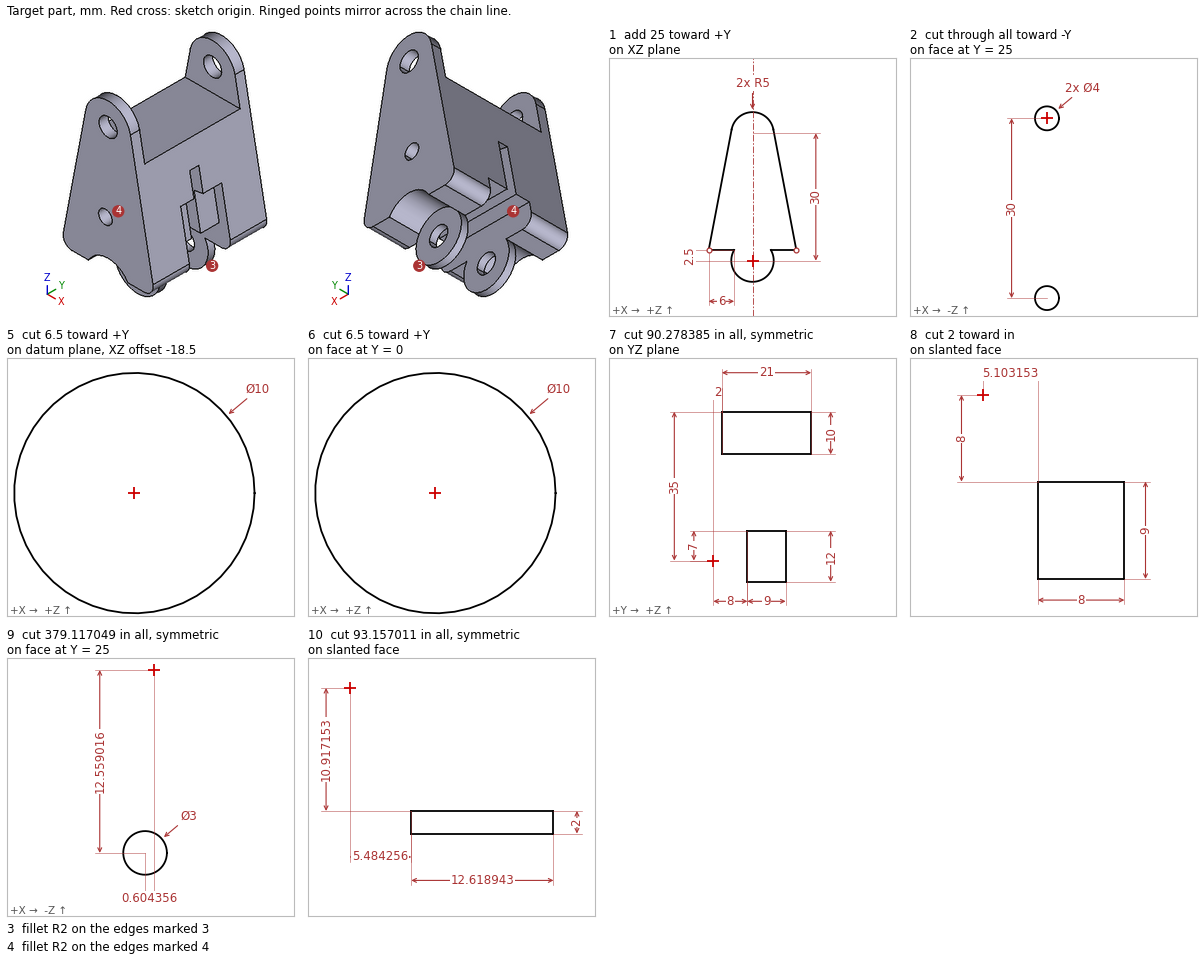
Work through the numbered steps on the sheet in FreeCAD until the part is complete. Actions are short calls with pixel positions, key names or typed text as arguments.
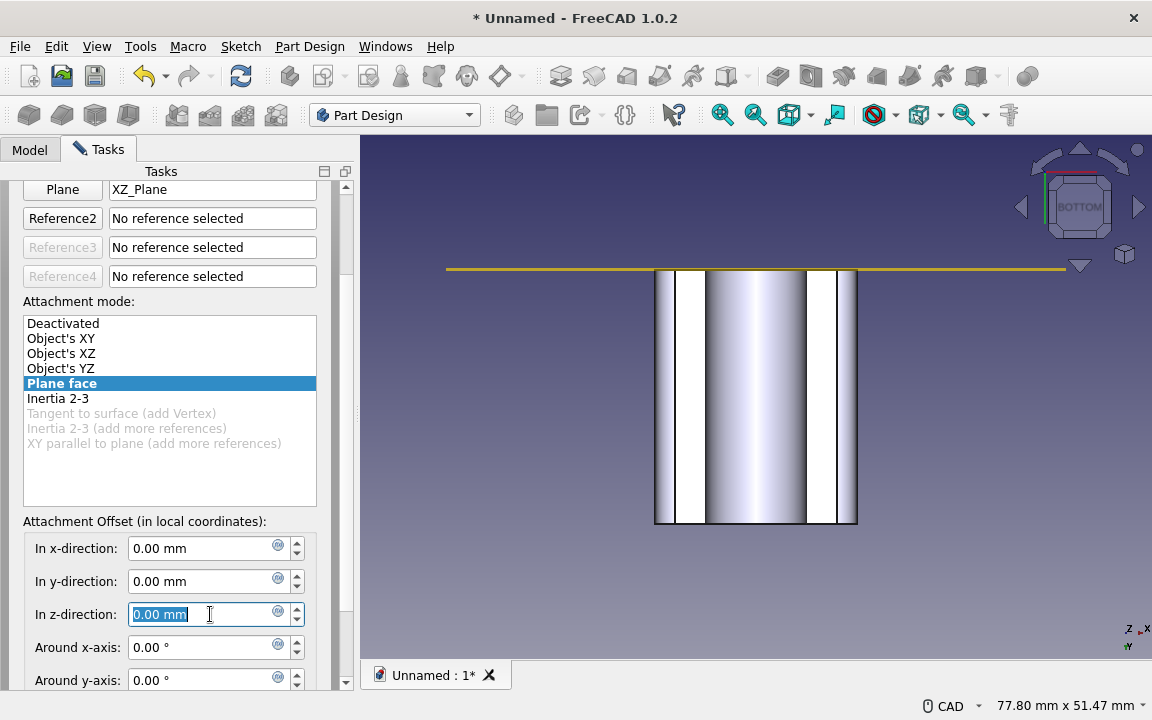
text(-18.5)
key(Tab)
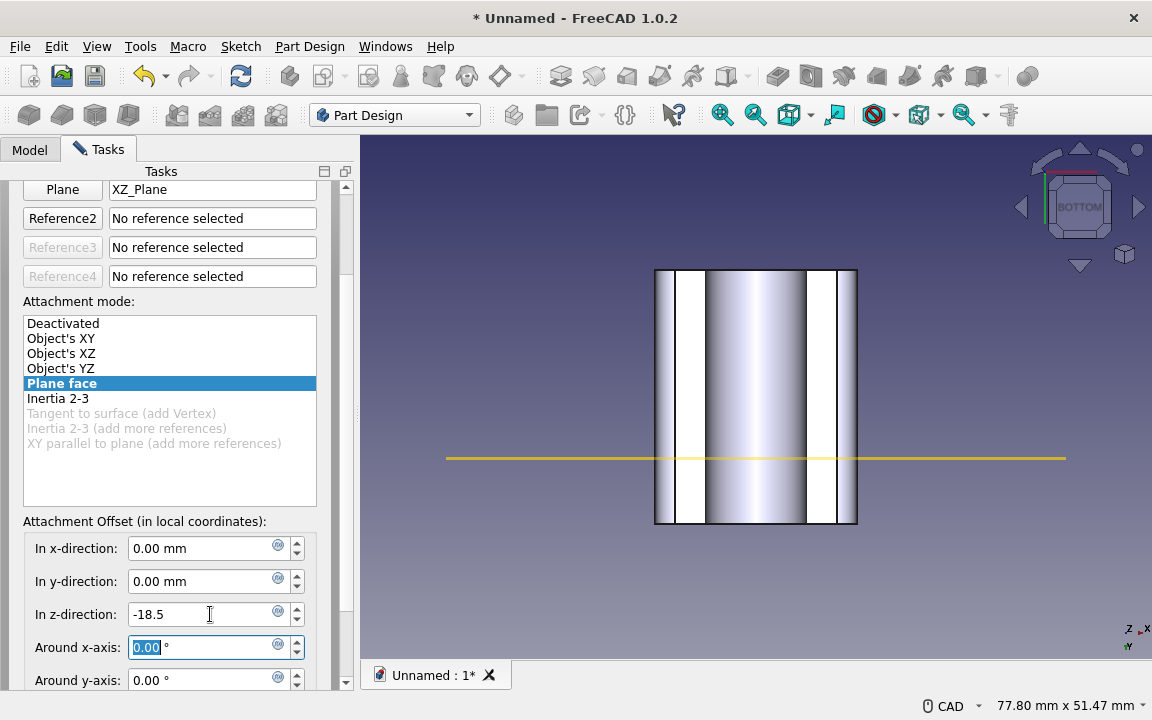
scroll(346, 436, up, 3)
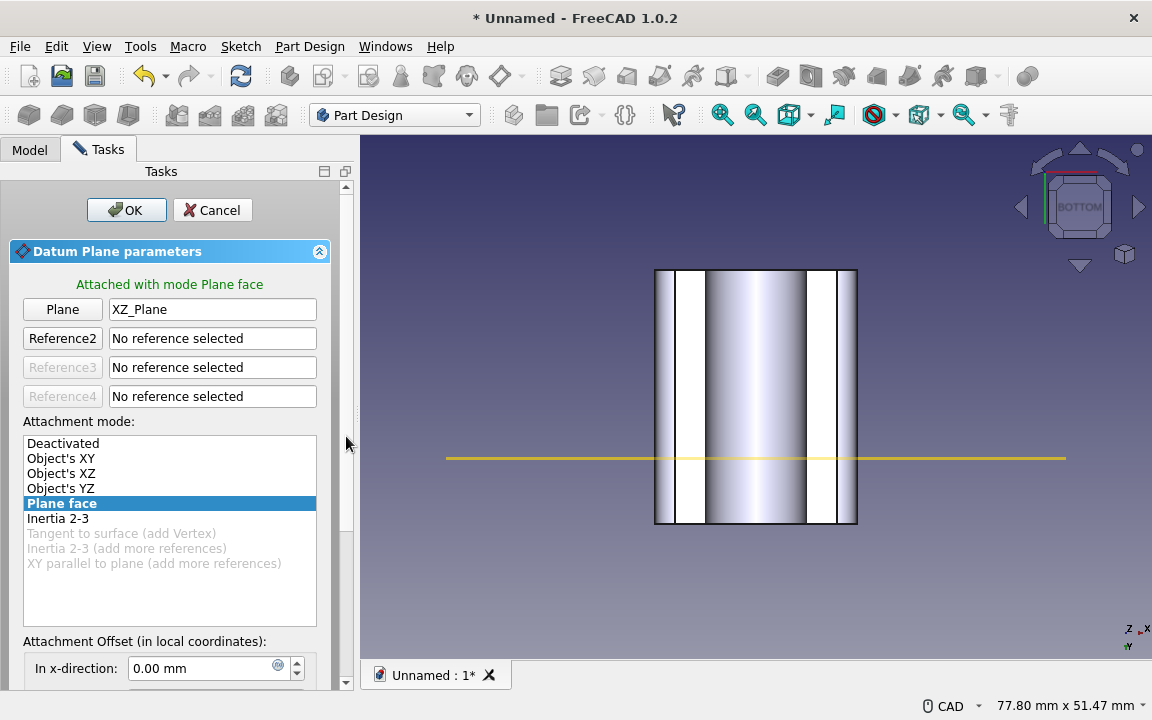
click(127, 210)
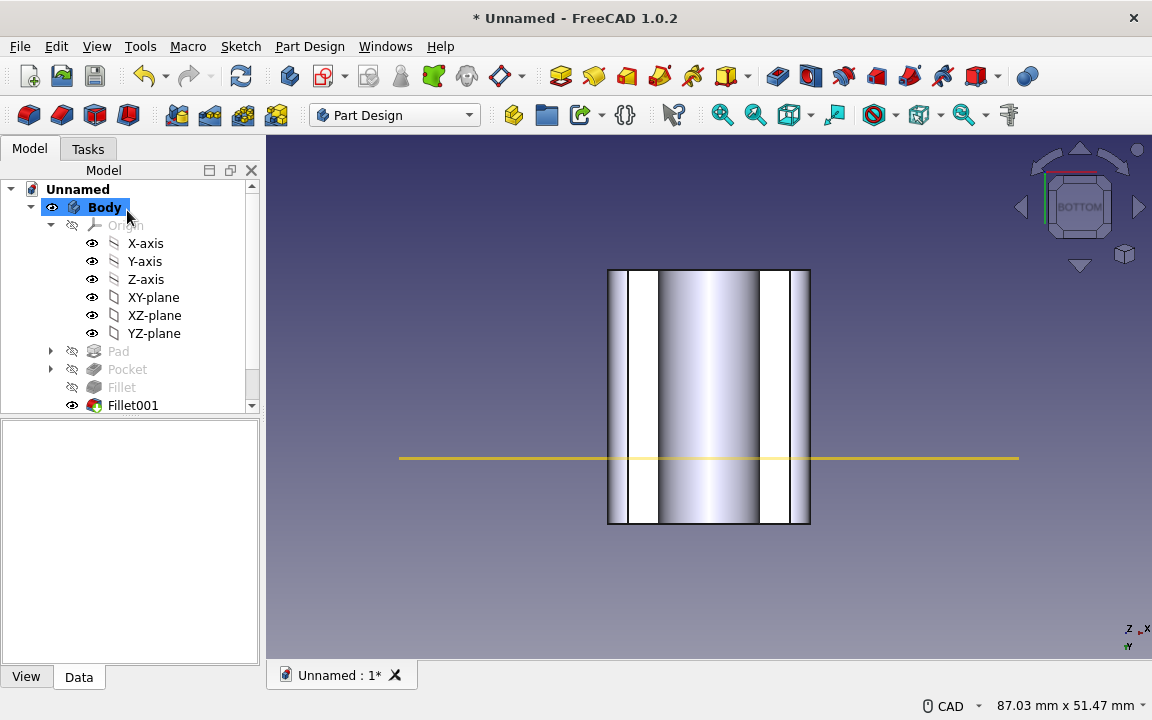
scroll(101, 293, down, 3)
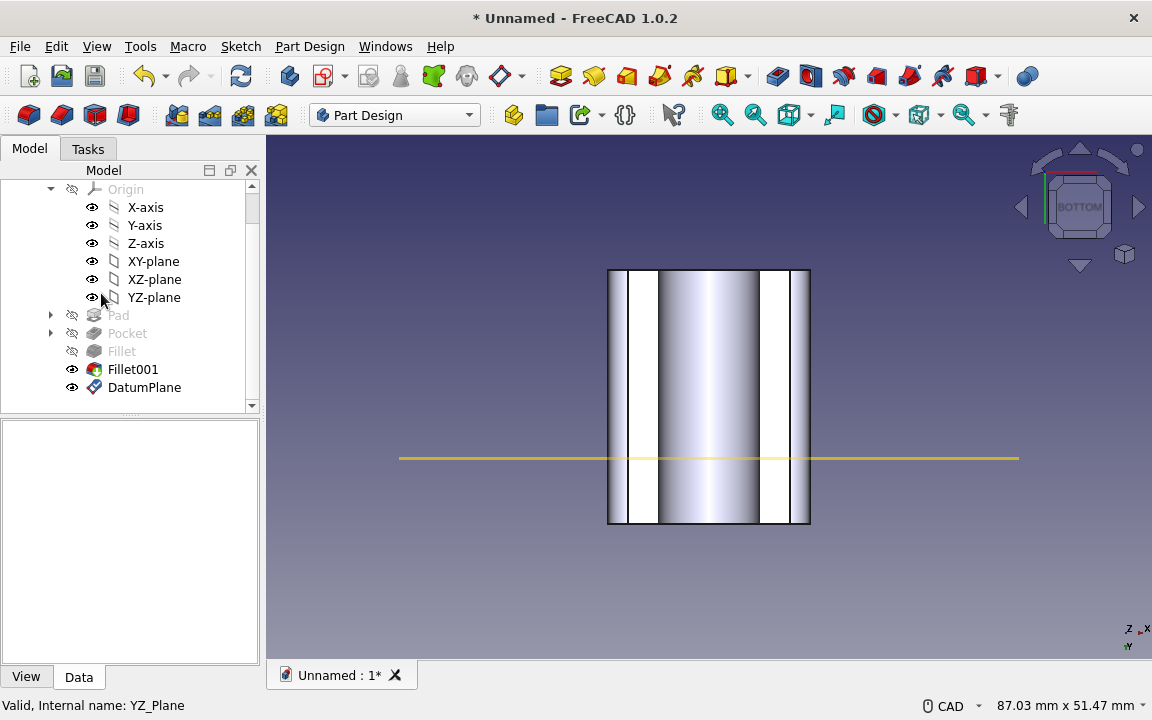
click(117, 387)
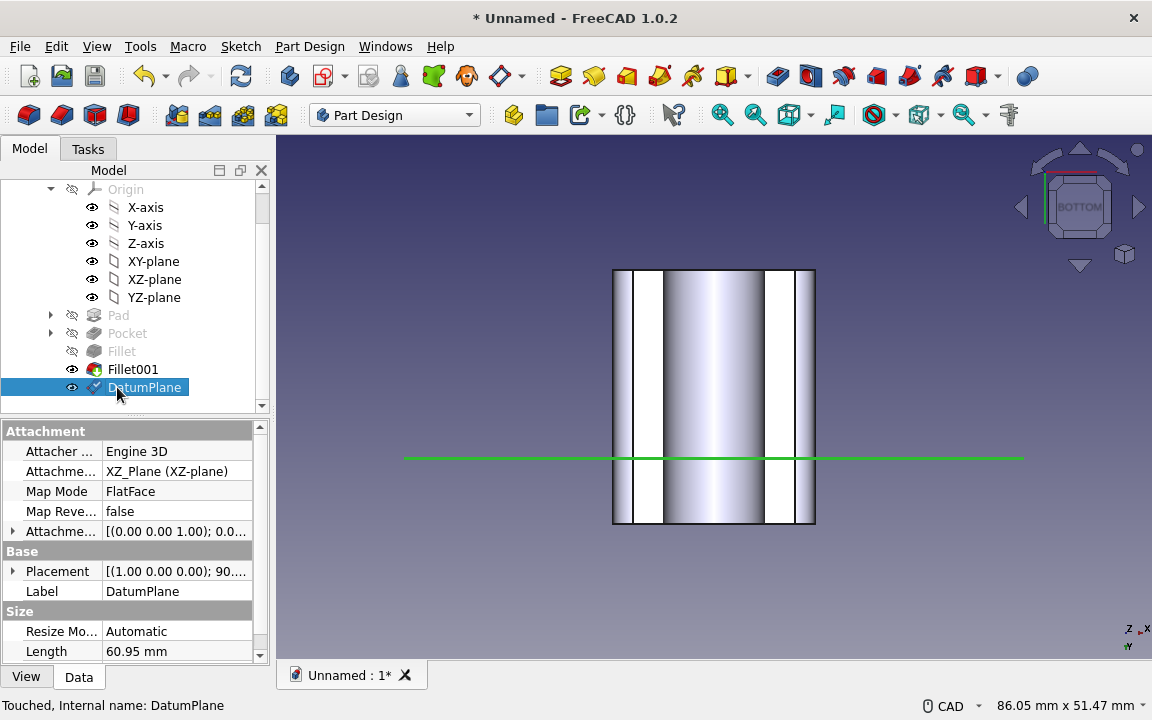
click(322, 76)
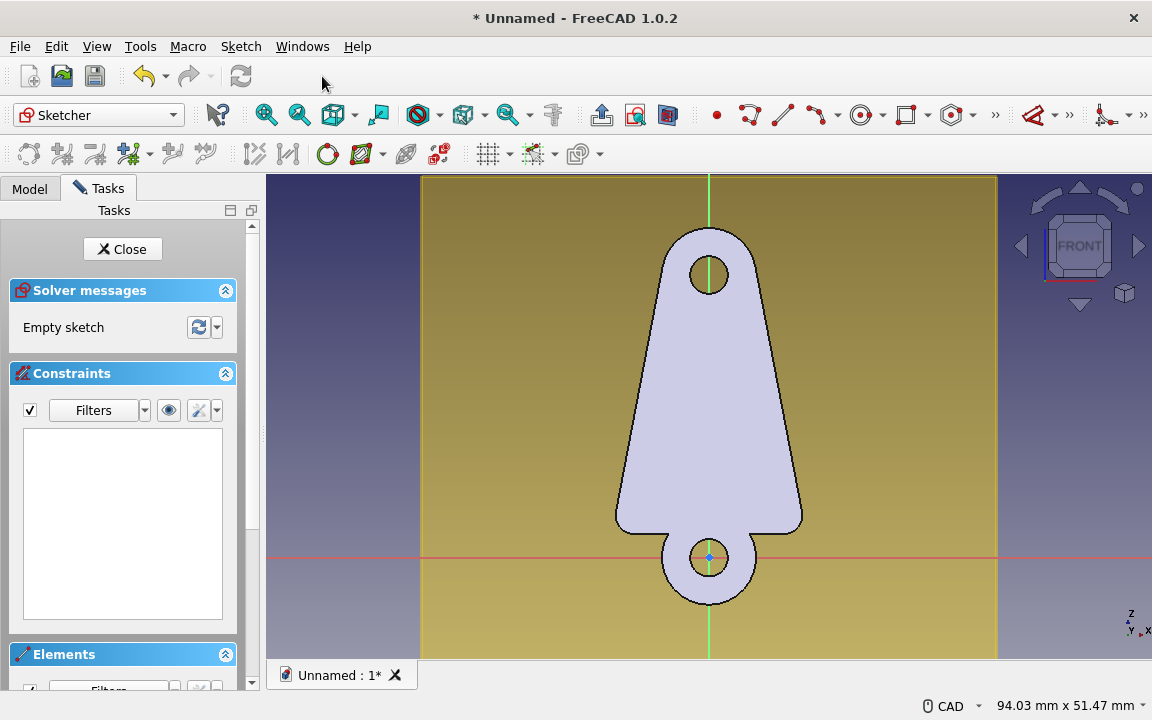
click(668, 116)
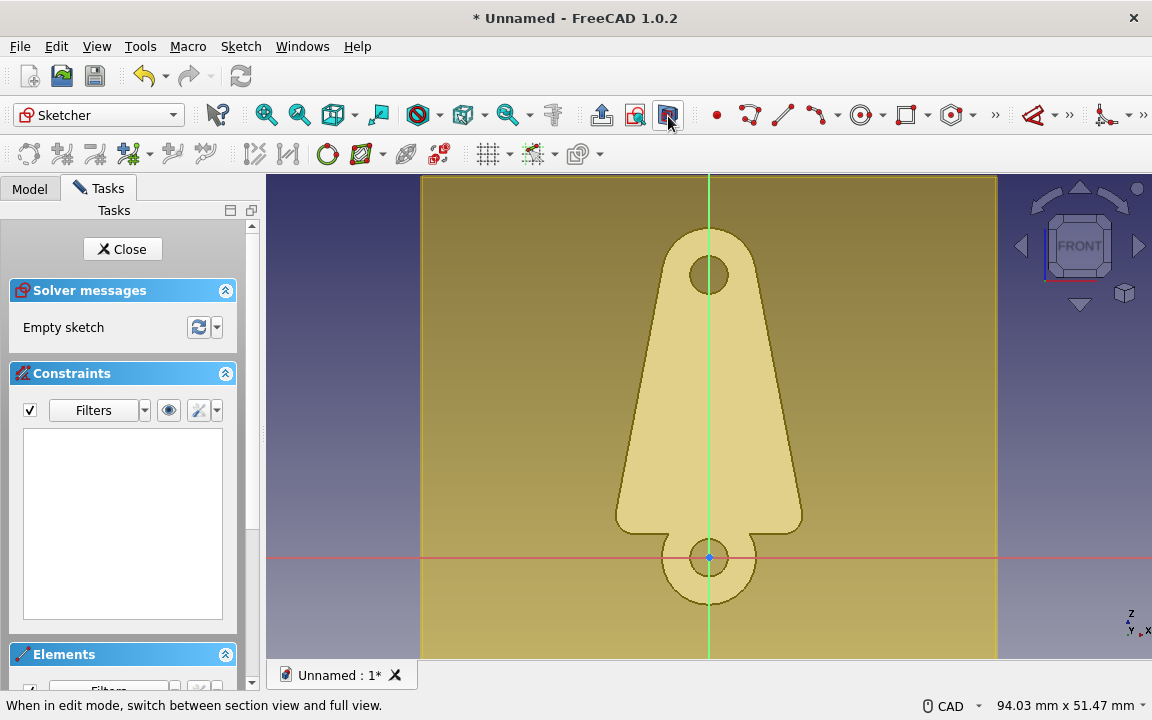
scroll(739, 619, up, 6)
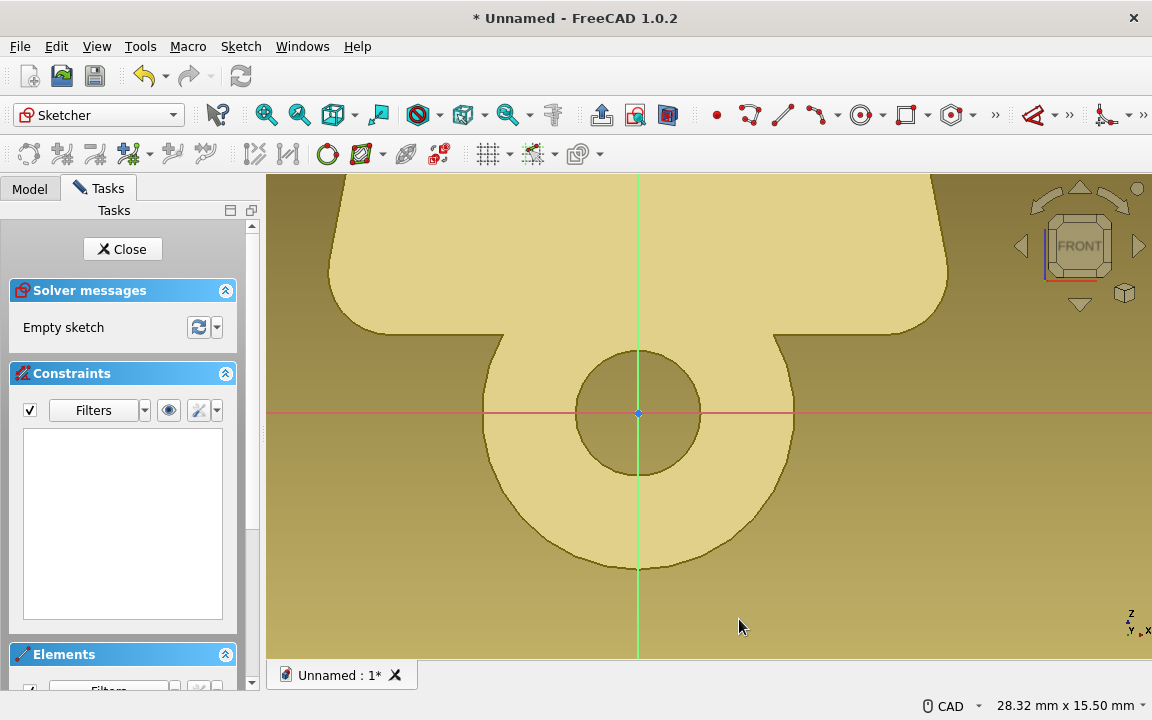
key(g)
key(c)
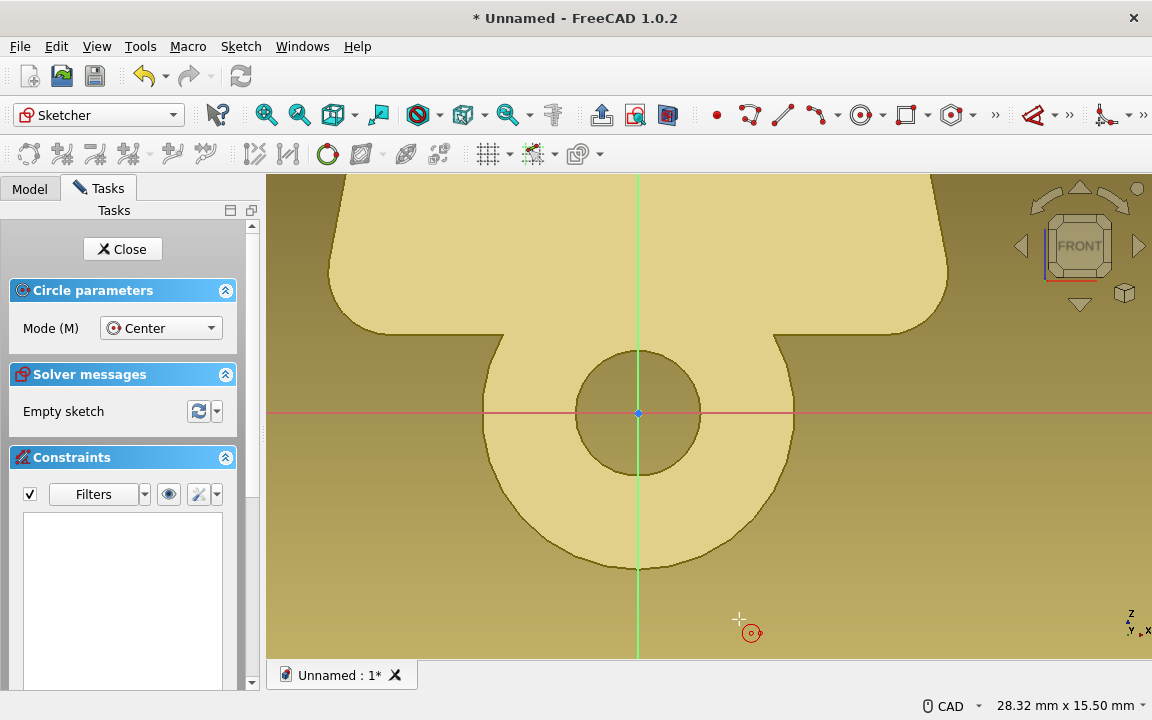
click(638, 413)
move(749, 303)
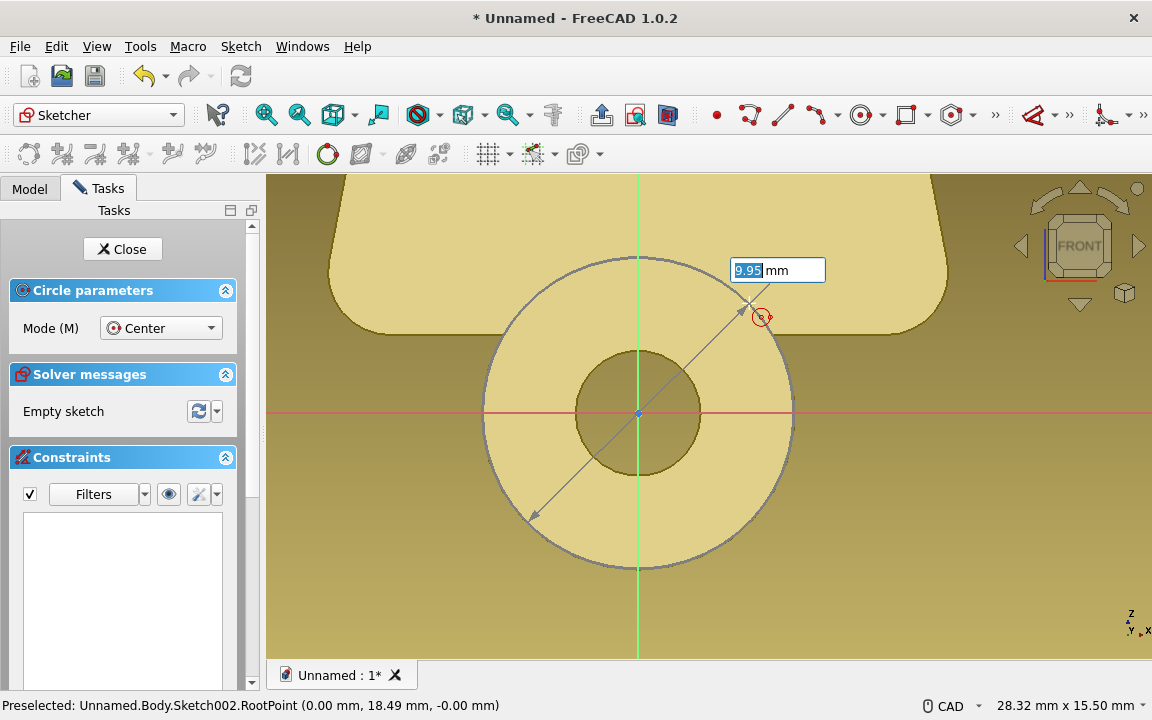
text(10)
key(Return)
key(Escape)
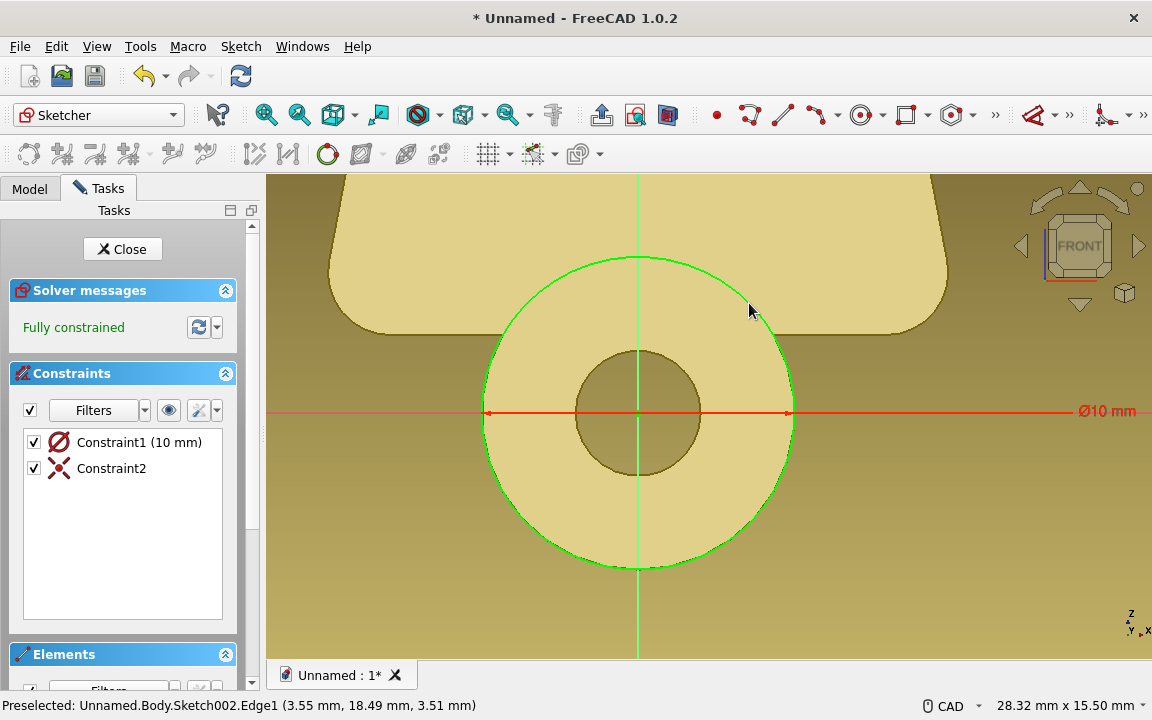
click(123, 249)